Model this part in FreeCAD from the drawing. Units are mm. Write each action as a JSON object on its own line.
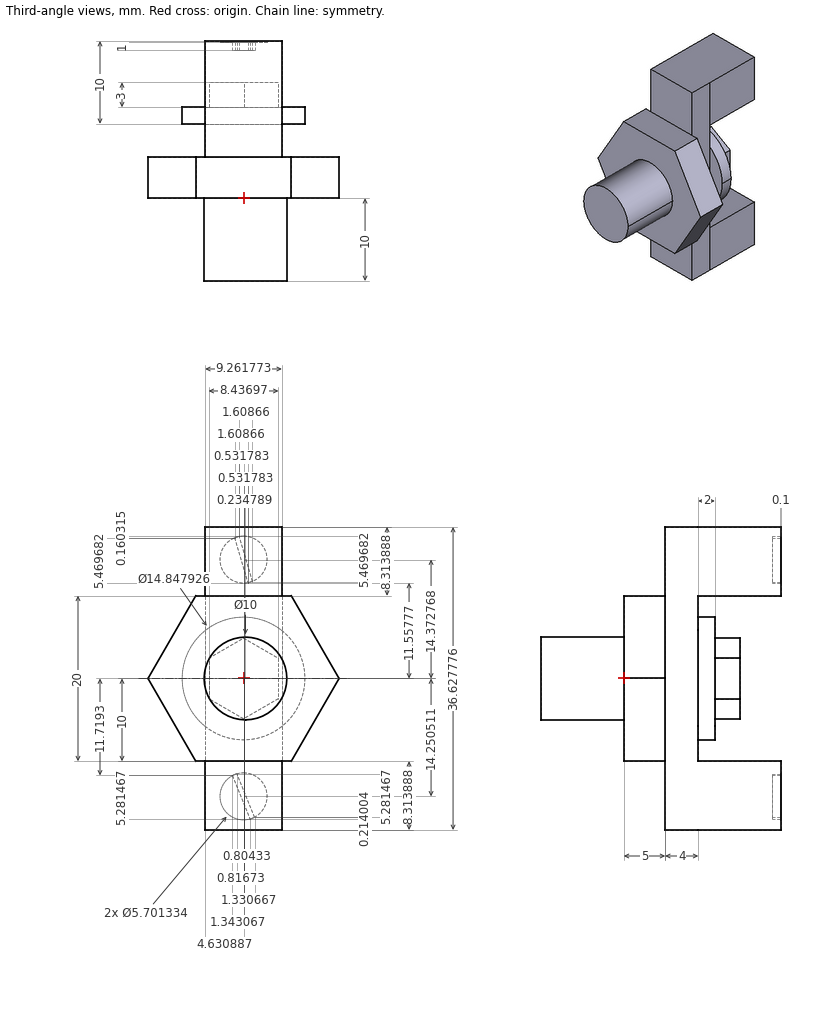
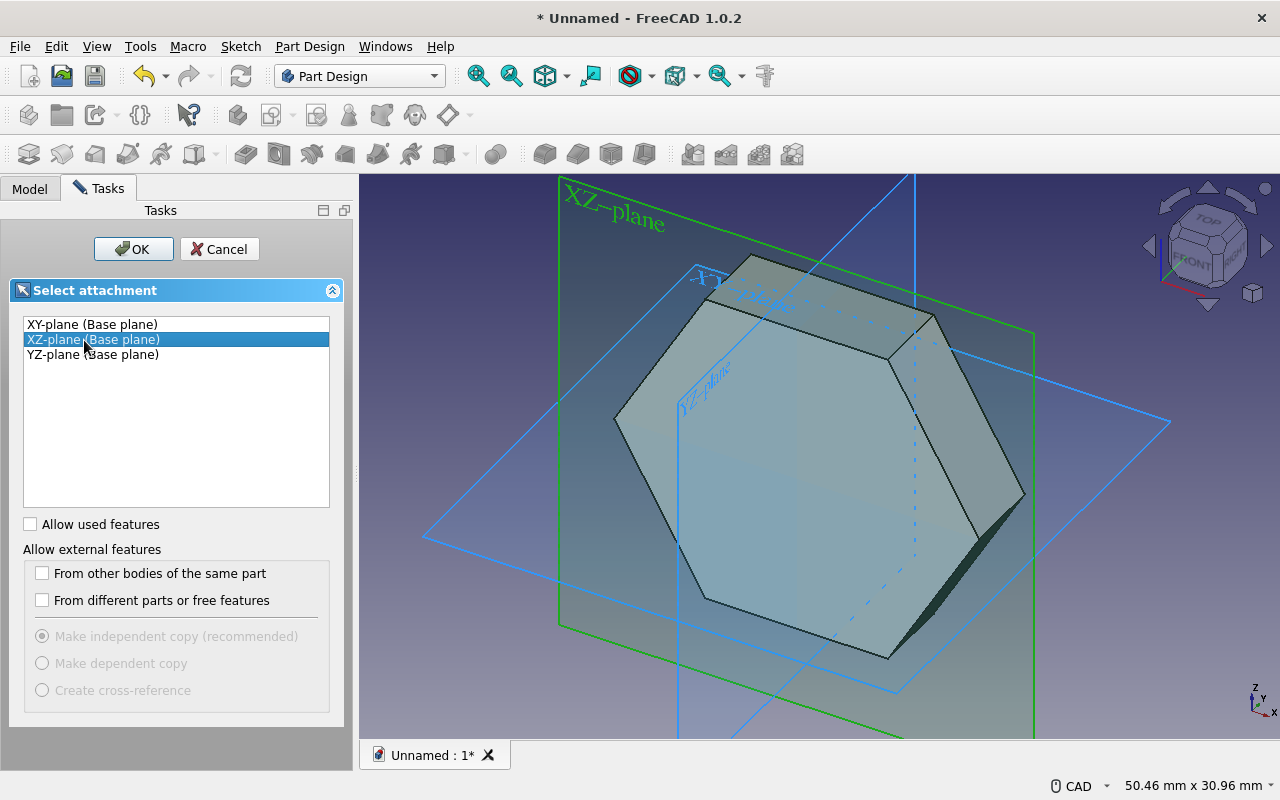
{"action": "left_click", "coordinate": [134, 249]}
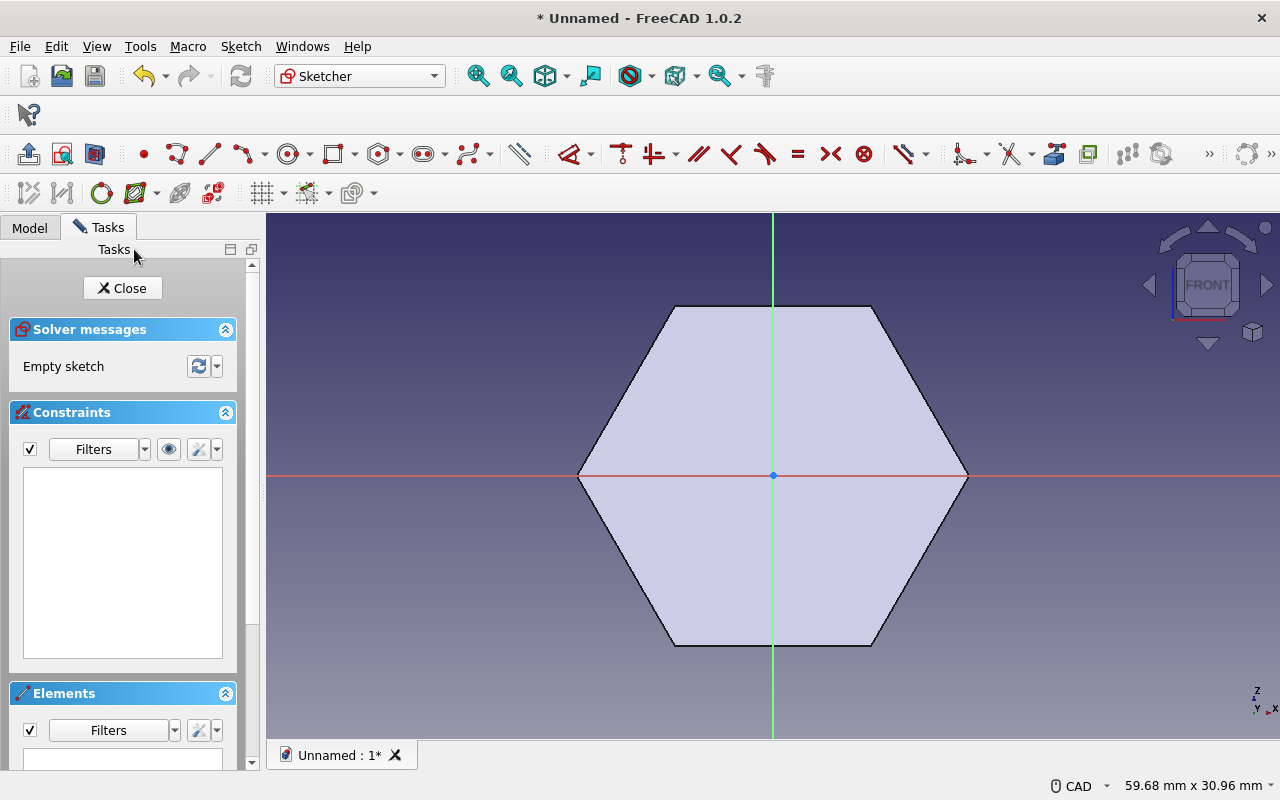
{"action": "scroll", "coordinate": [865, 476], "scroll_direction": "up", "scroll_amount": 3}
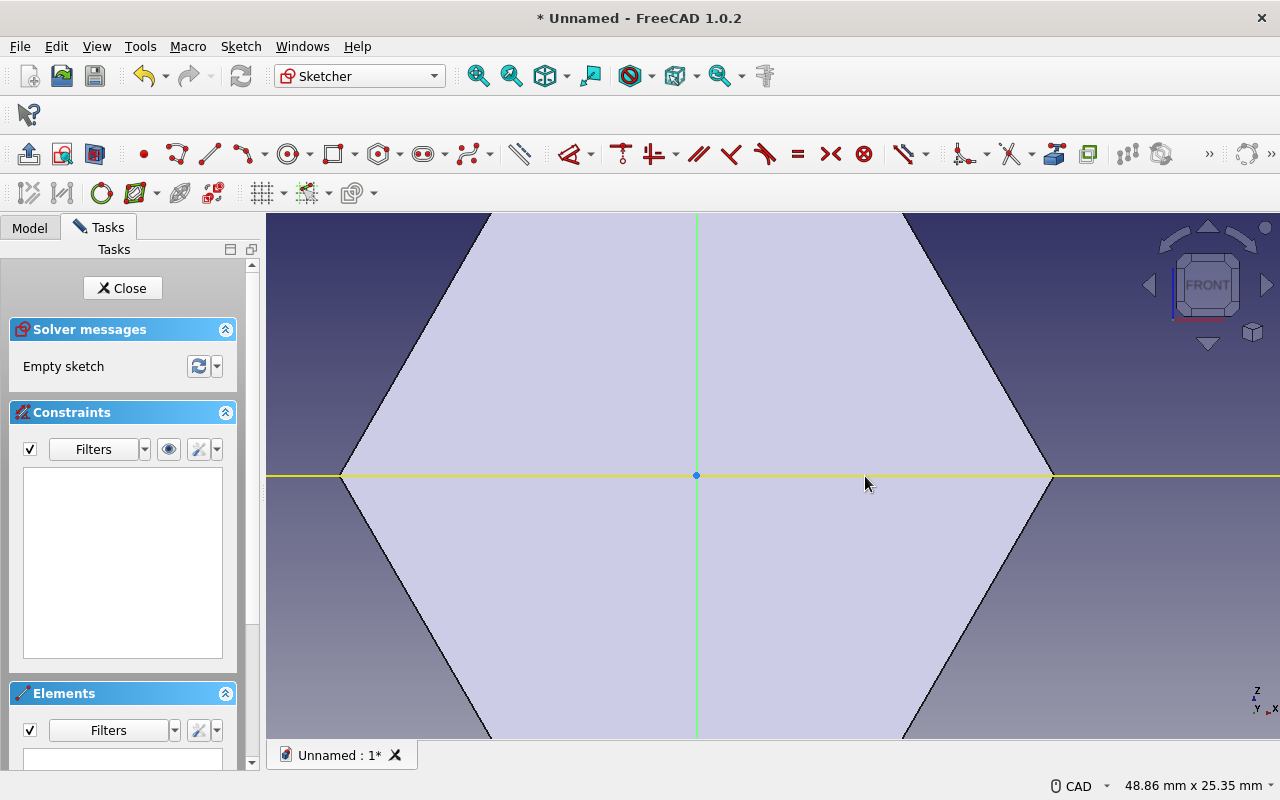
{"action": "left_click", "coordinate": [288, 154]}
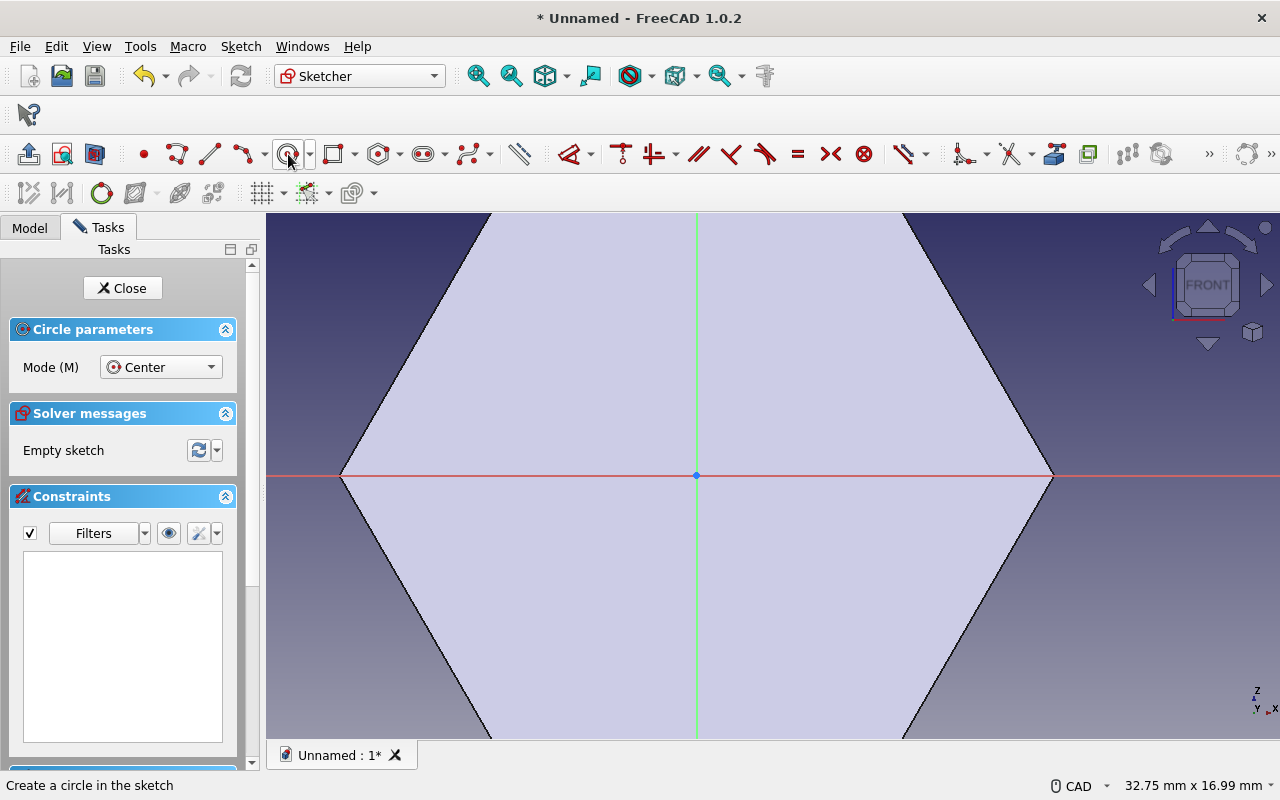
{"action": "scroll", "coordinate": [704, 476], "scroll_direction": "up", "scroll_amount": 4}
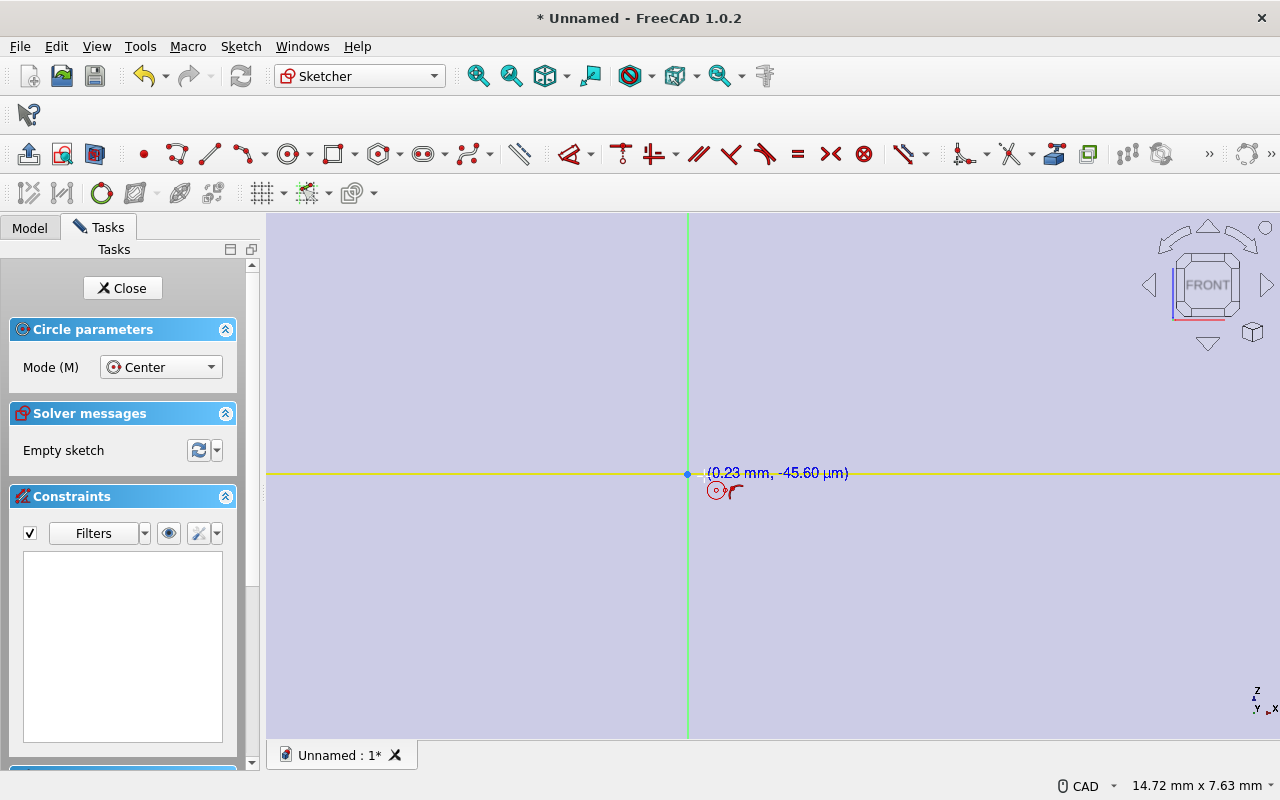
{"action": "left_click", "coordinate": [704, 474]}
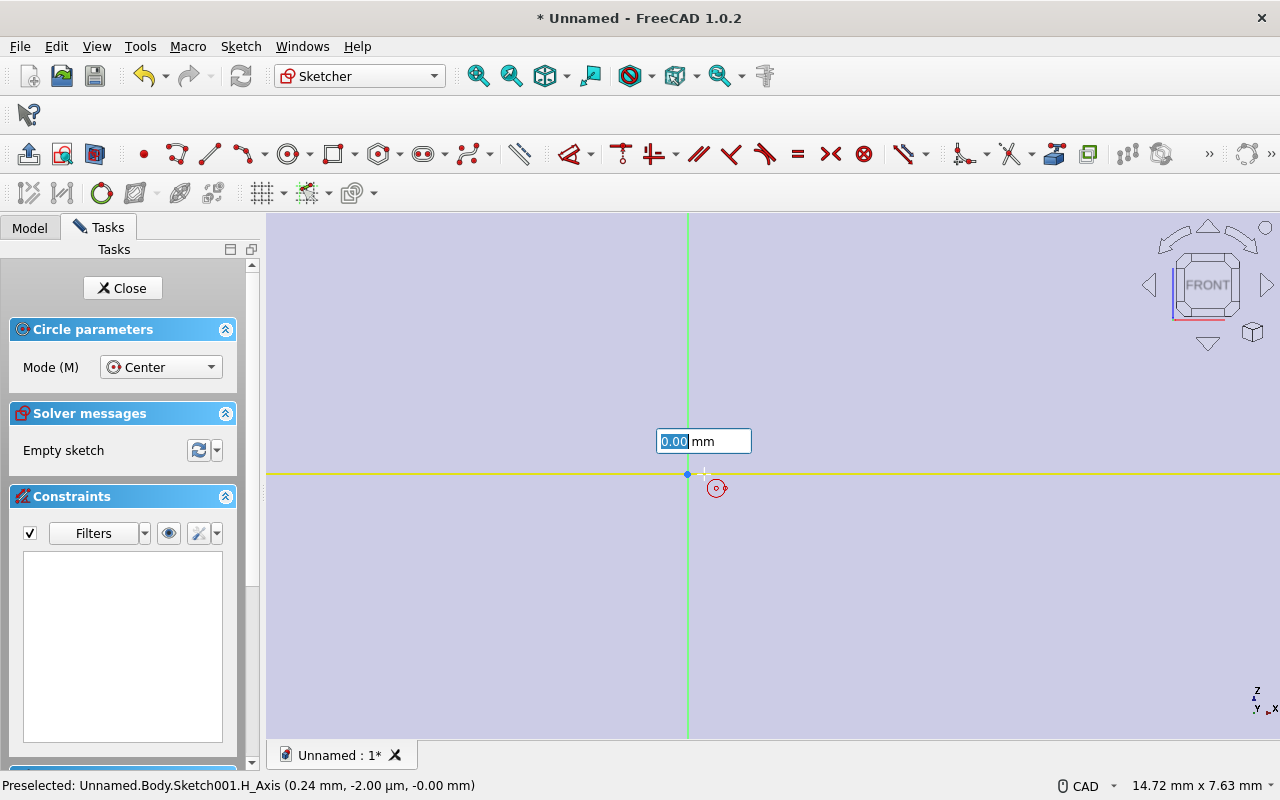
{"action": "scroll", "coordinate": [705, 477], "scroll_direction": "down", "scroll_amount": 4}
{"action": "mouse_move", "coordinate": [814, 367]}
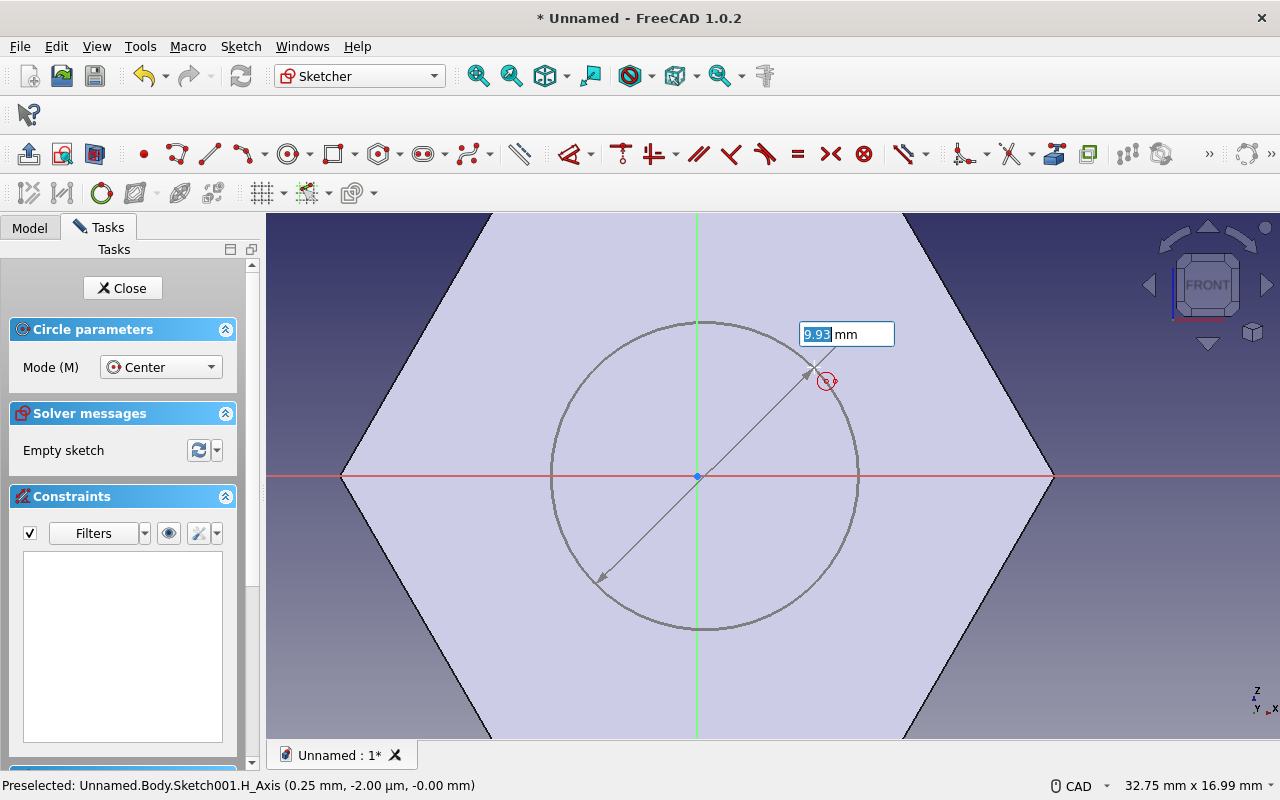
{"action": "type", "text": "10"}
{"action": "key", "text": "Return"}
{"action": "key", "text": "Escape"}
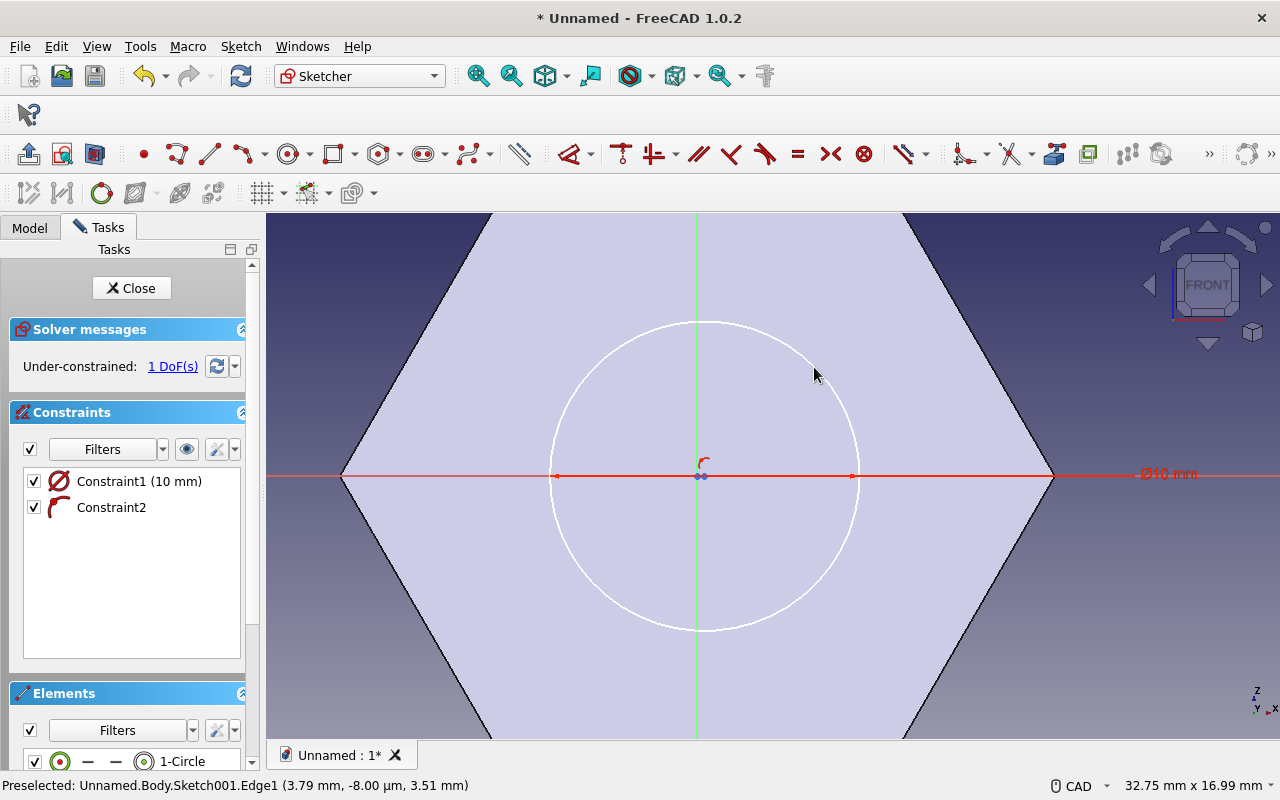
{"action": "left_click", "coordinate": [568, 154]}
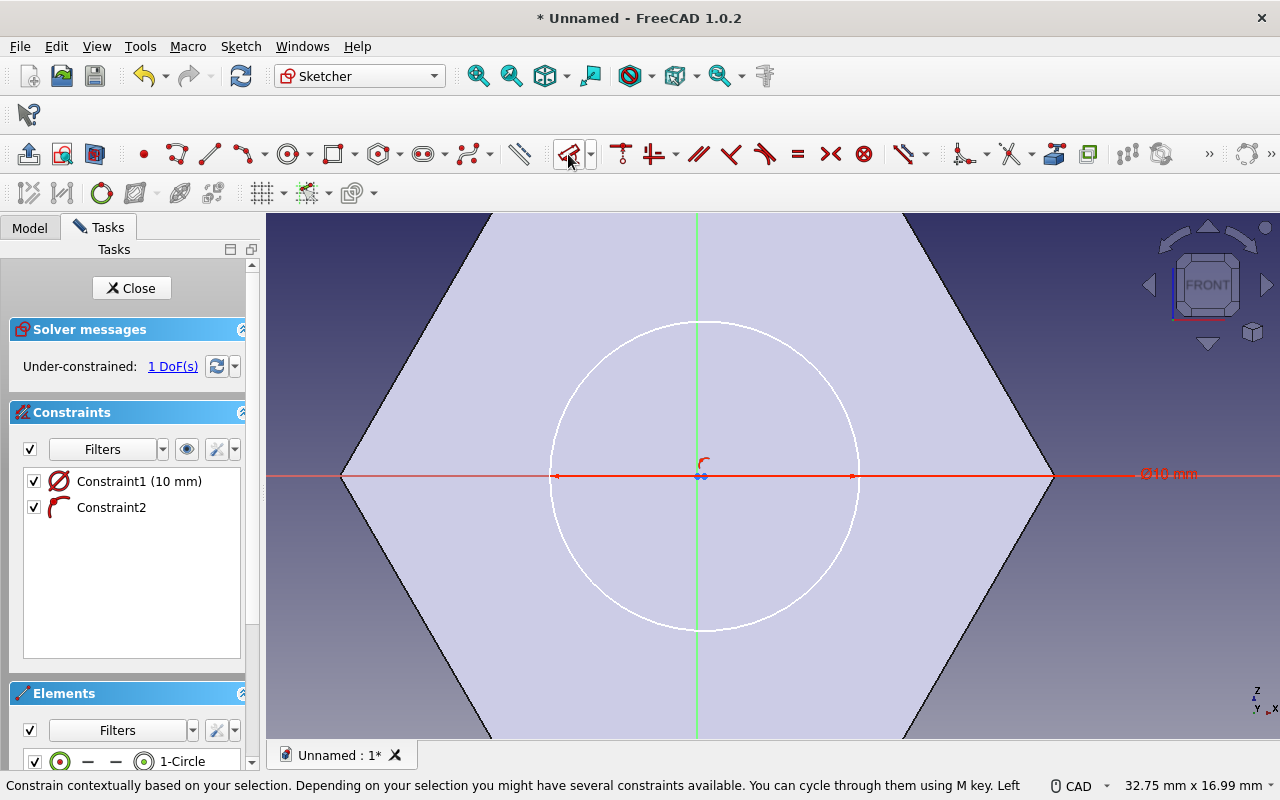
{"action": "scroll", "coordinate": [705, 476], "scroll_direction": "up", "scroll_amount": 9}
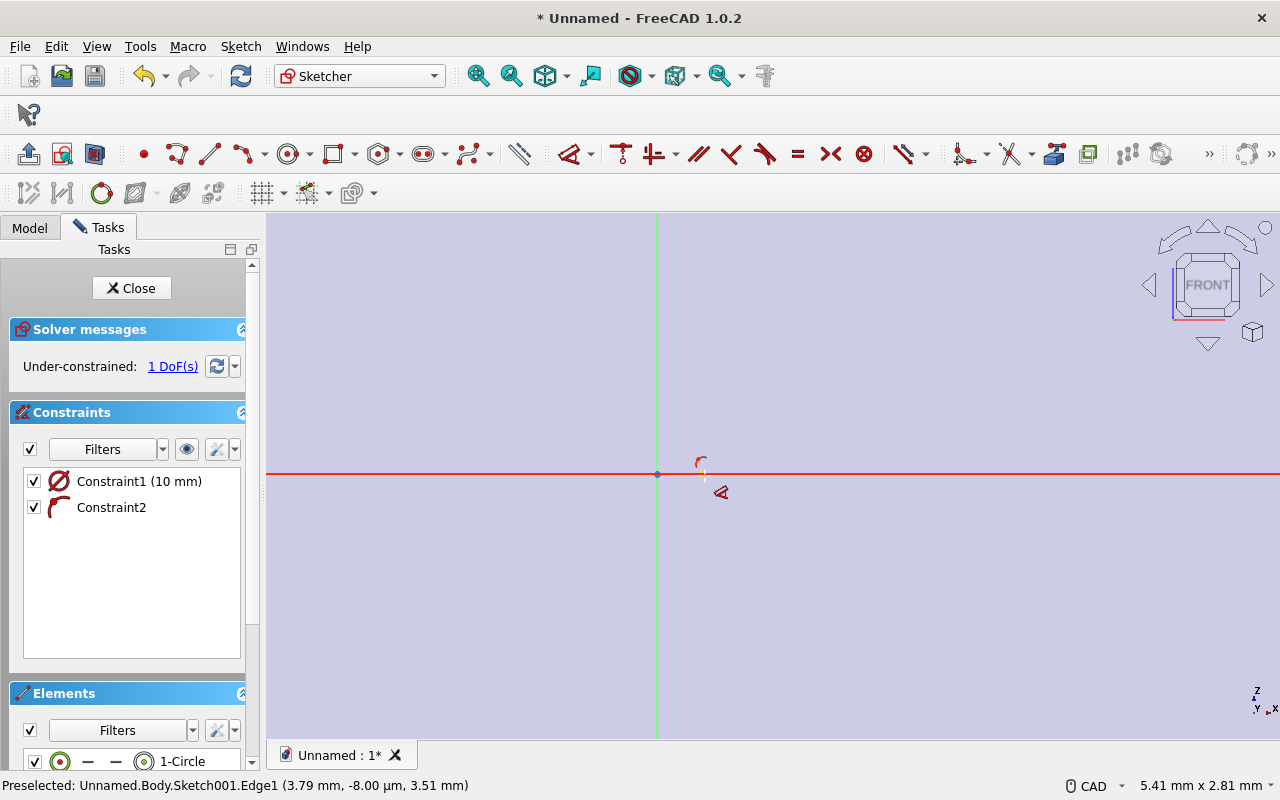
{"action": "left_click", "coordinate": [702, 474]}
{"action": "left_click", "coordinate": [679, 508]}